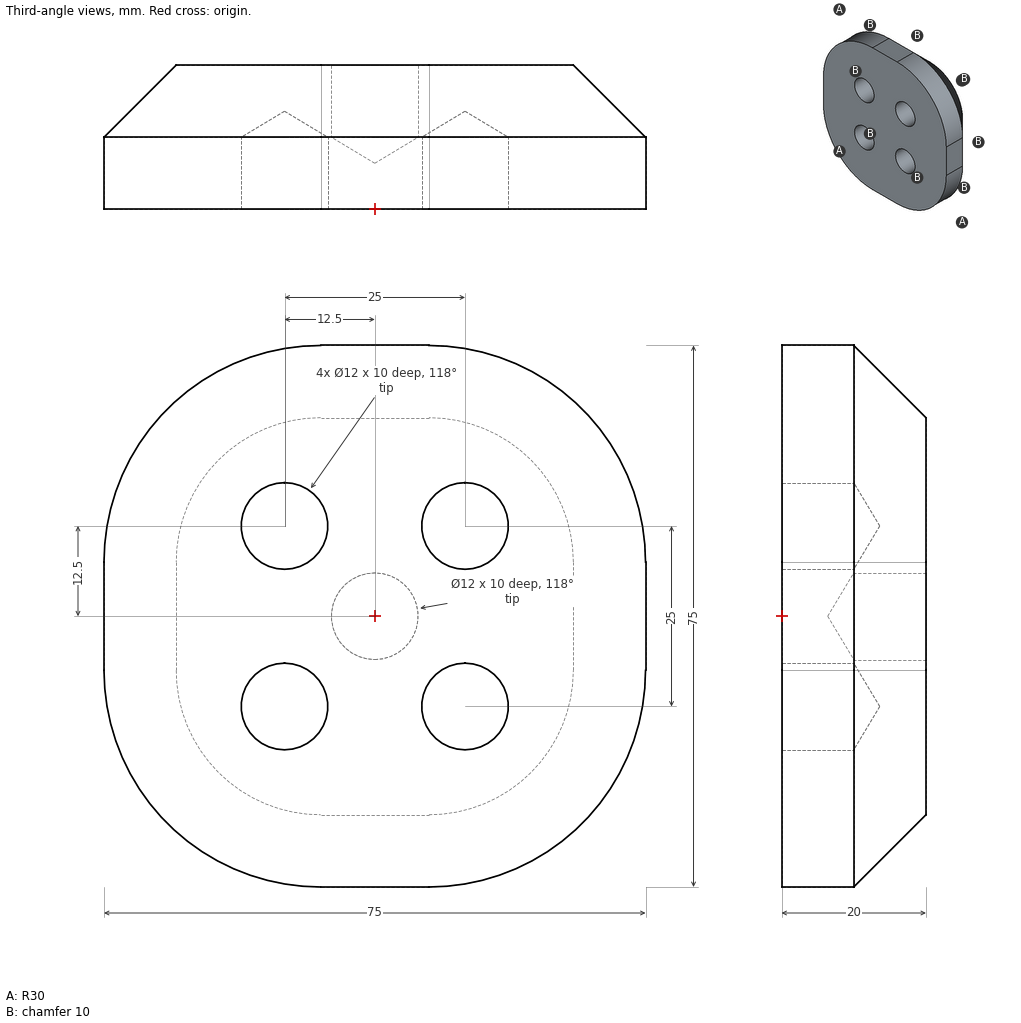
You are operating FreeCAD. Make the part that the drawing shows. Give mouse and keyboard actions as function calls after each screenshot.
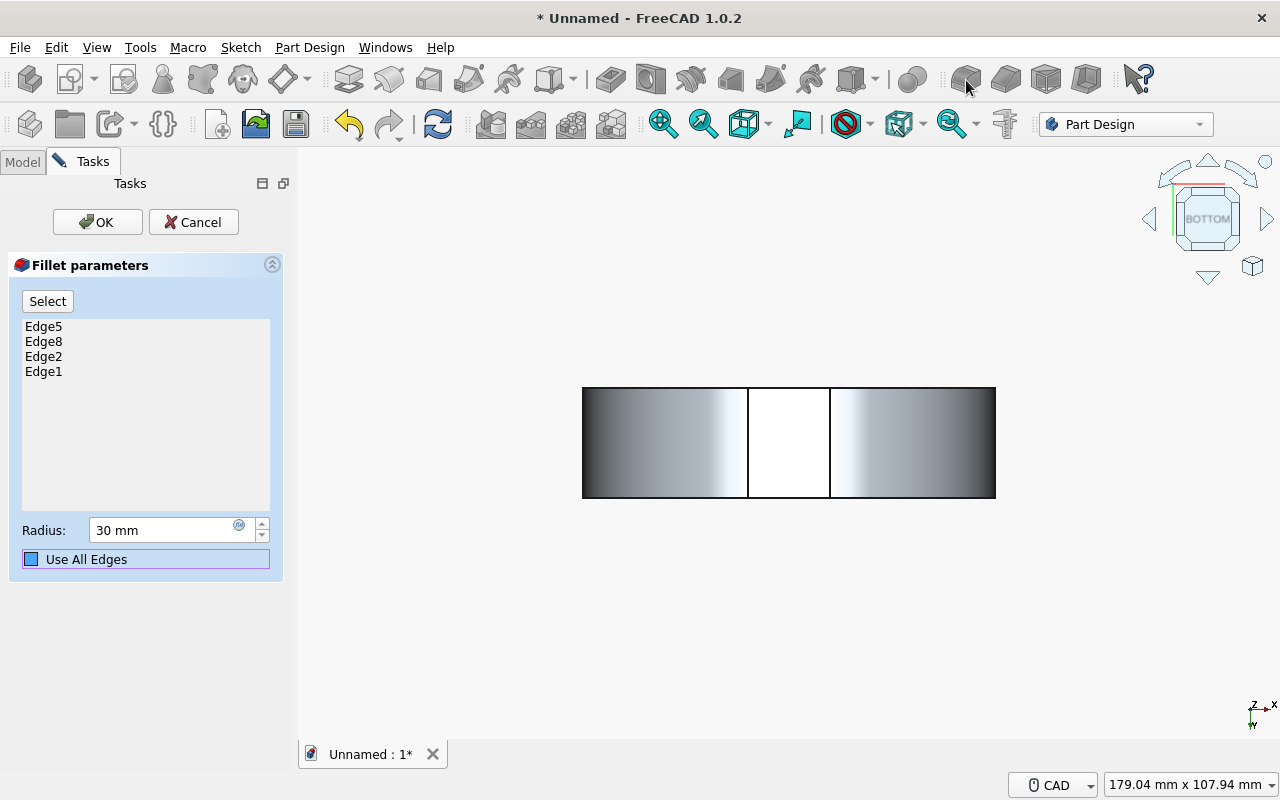
click(98, 222)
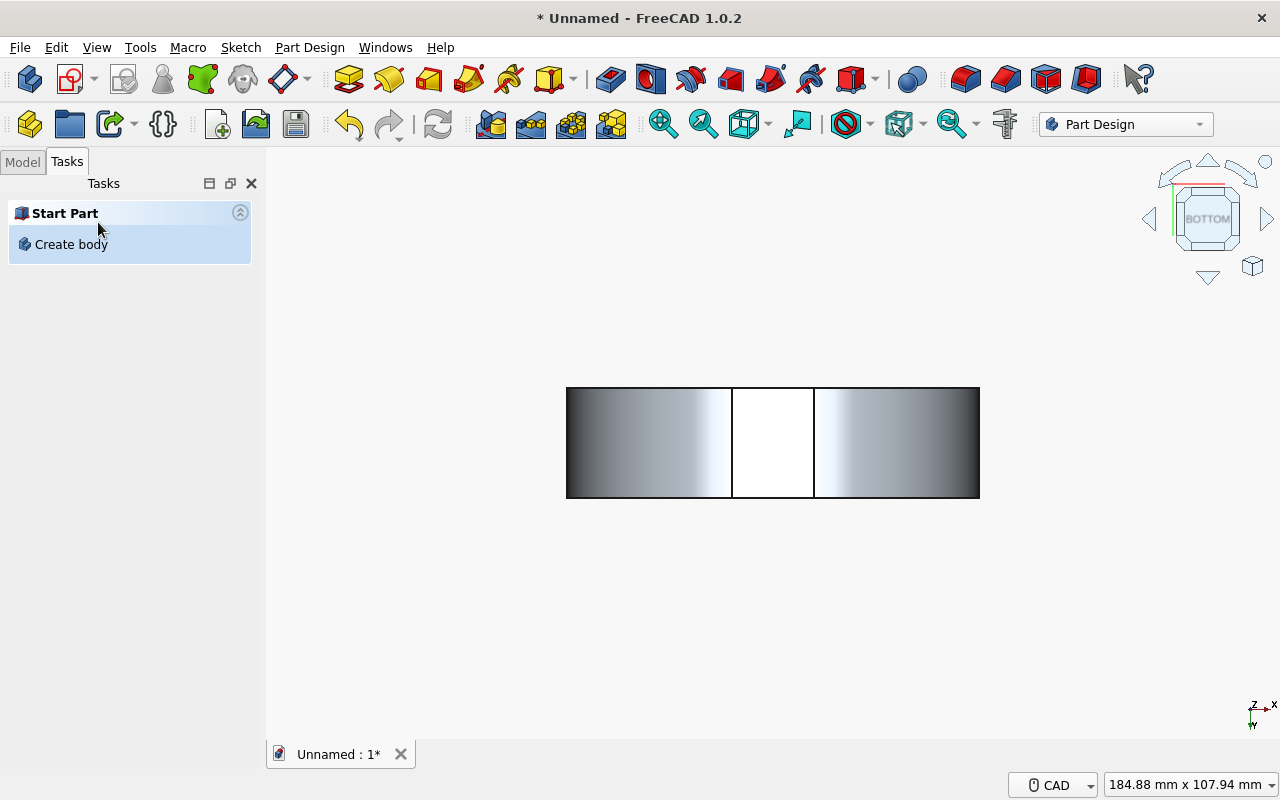
key(v)
key(f)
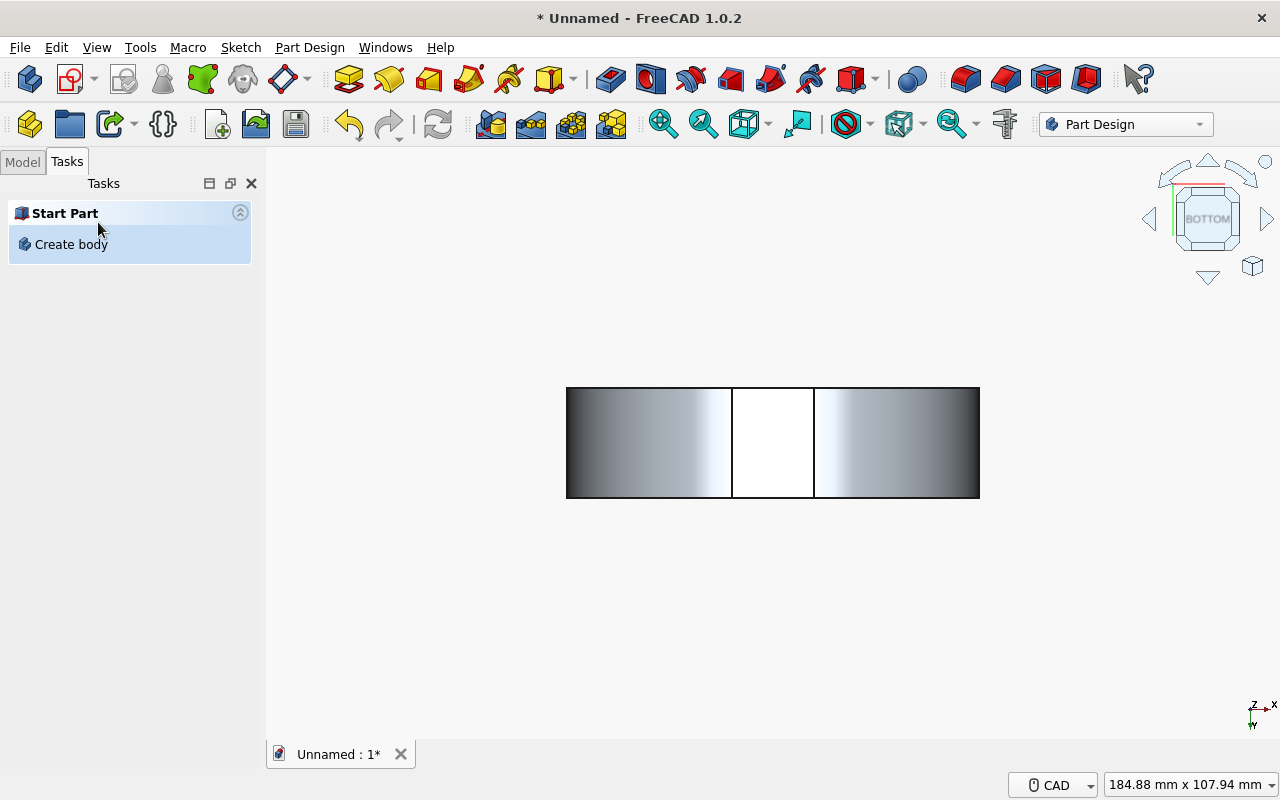
key(0)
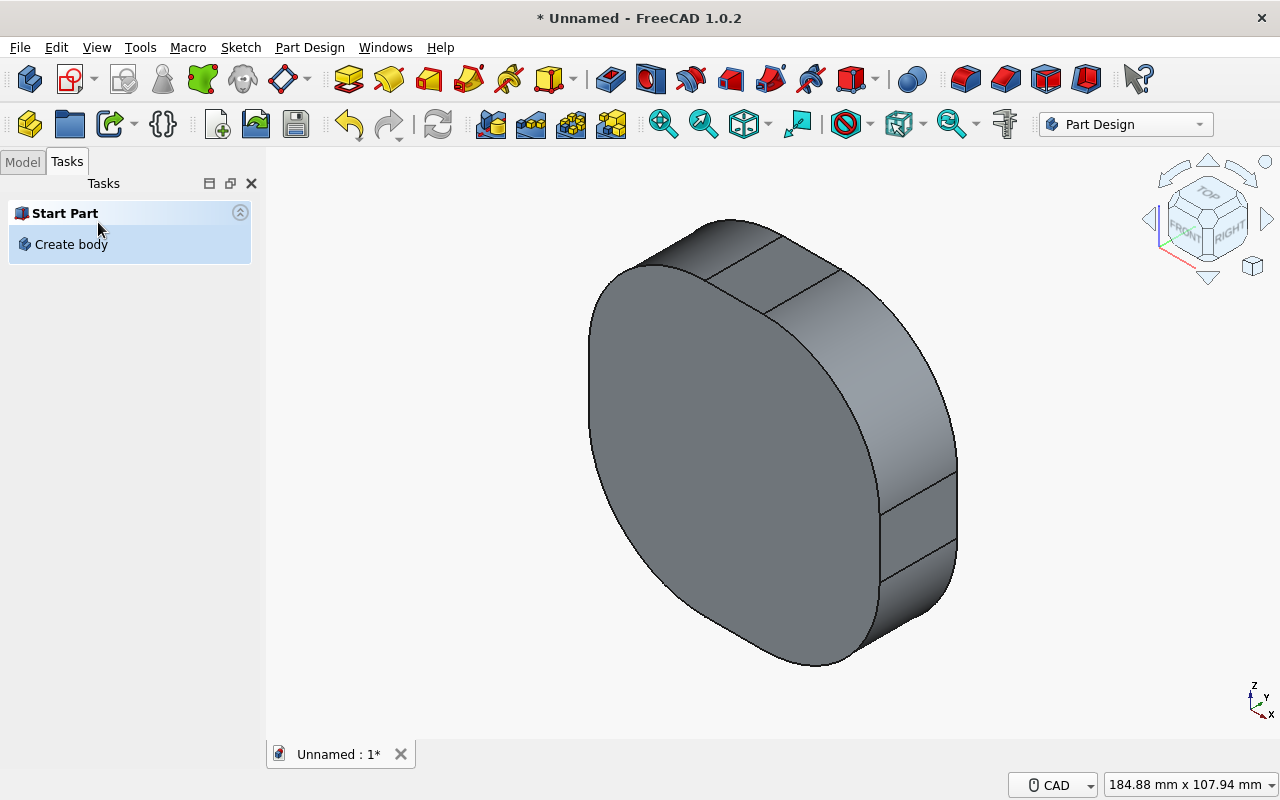
key(2)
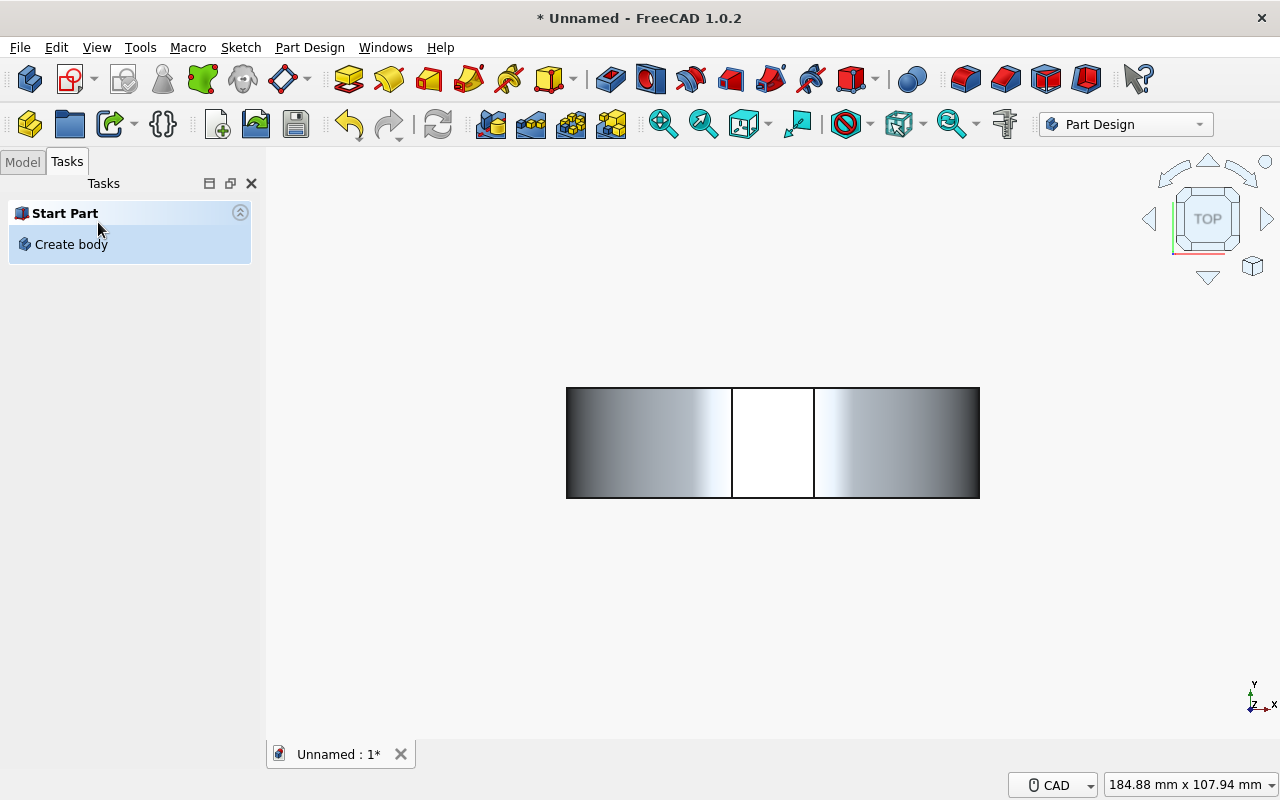
key(v)
key(f)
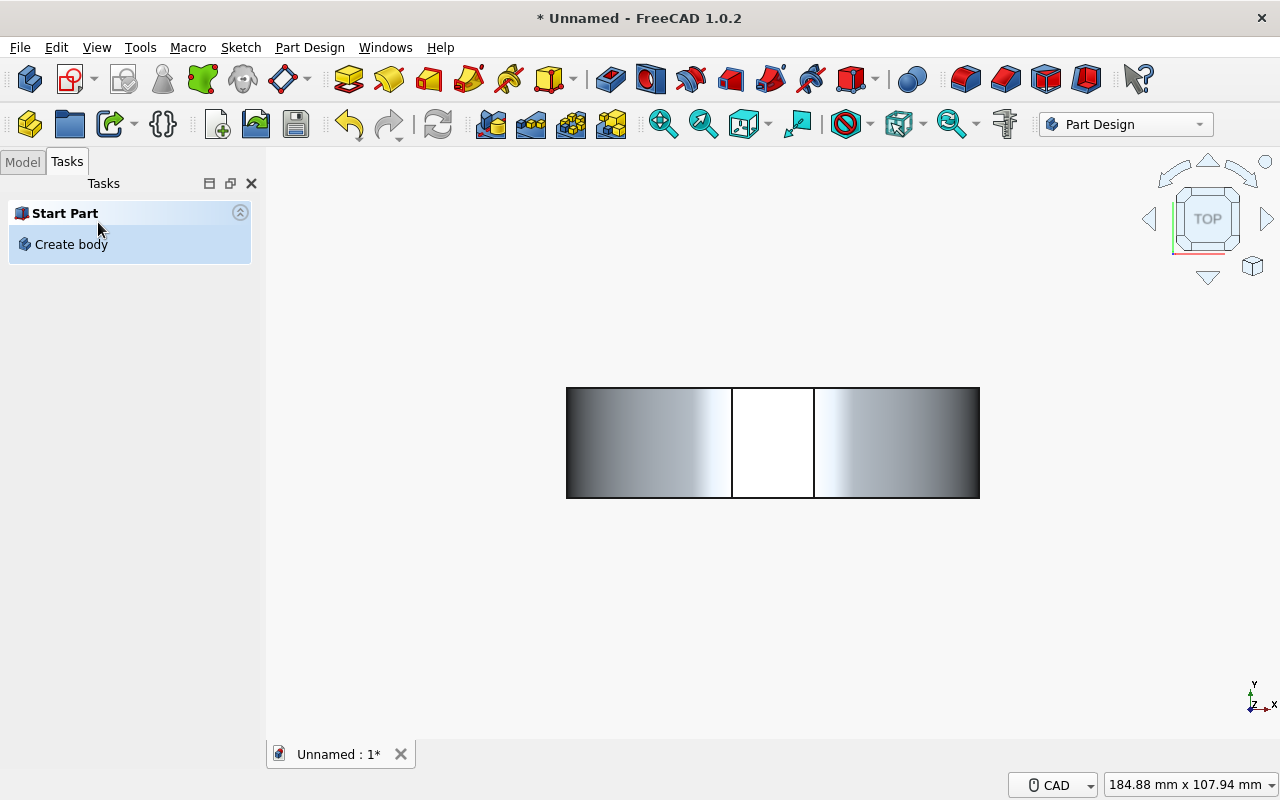
key(1)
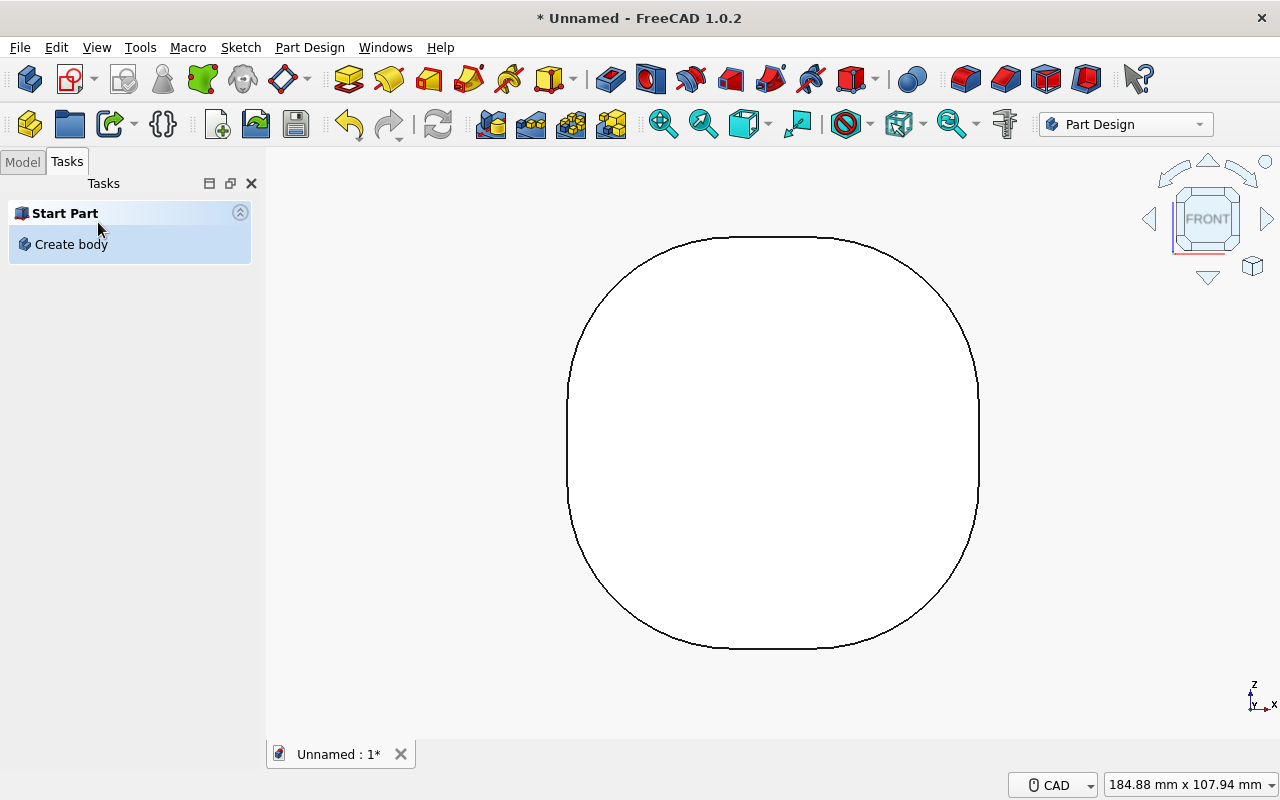
key(3)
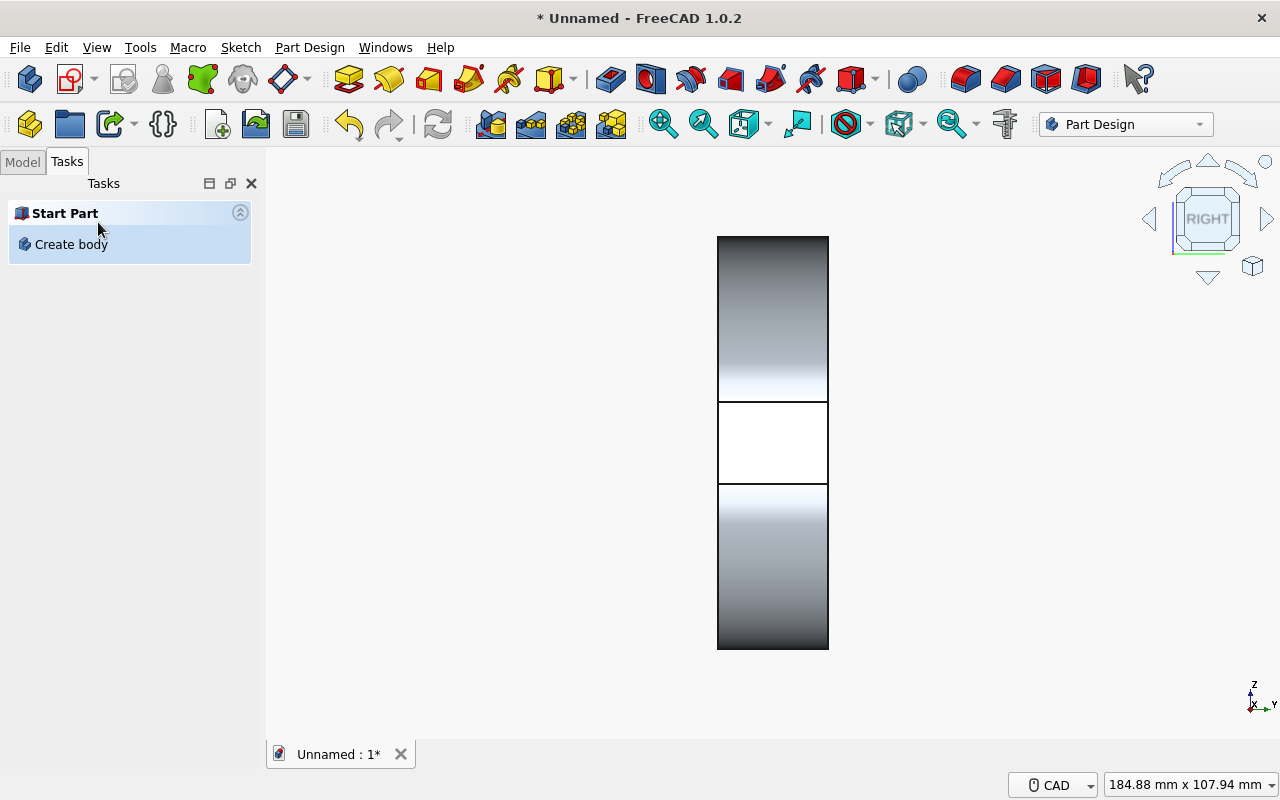
key(5)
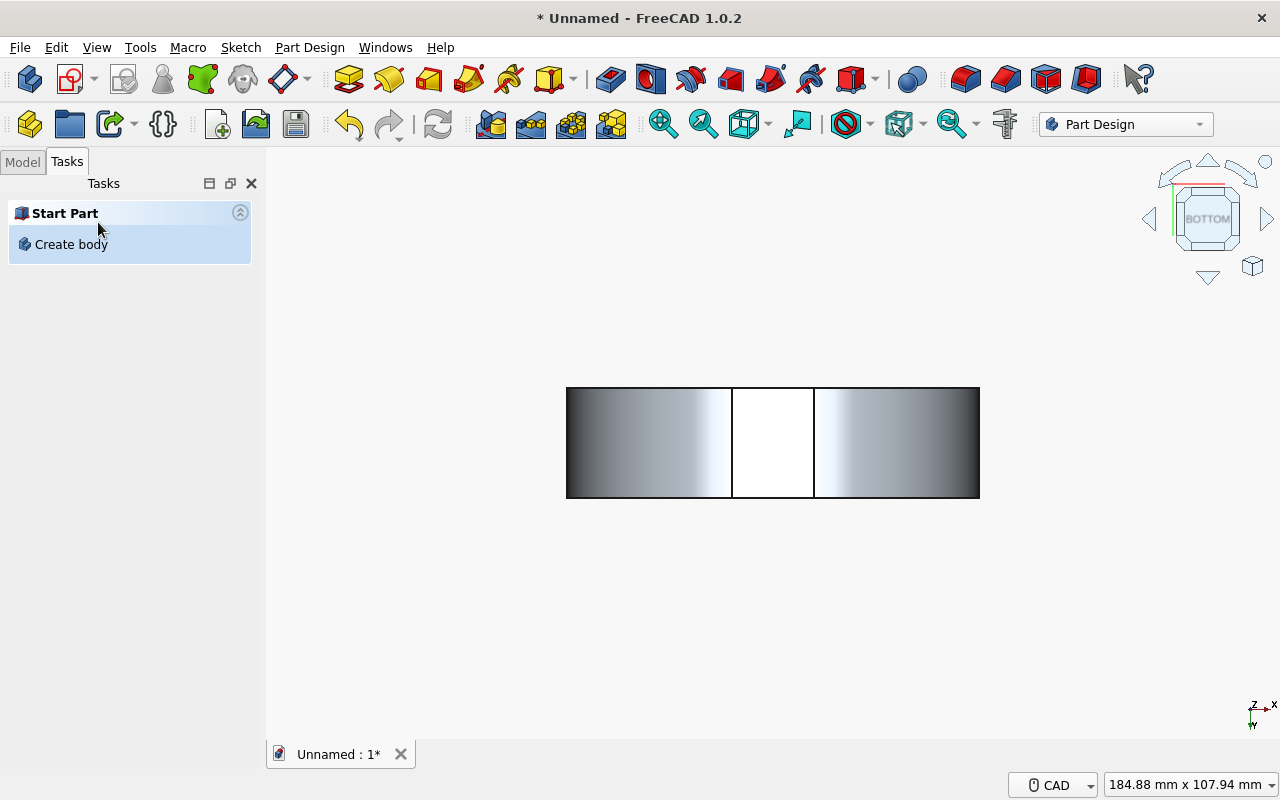
click(664, 124)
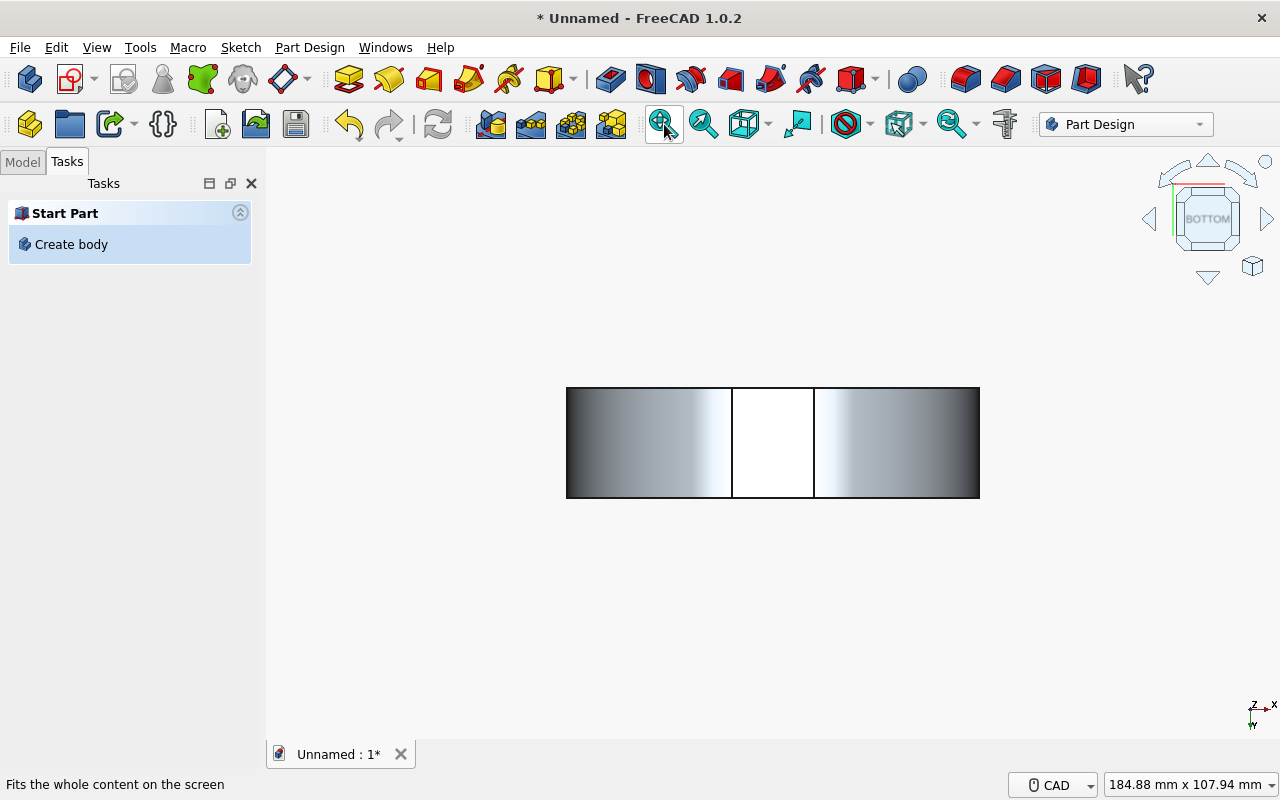
key(4)